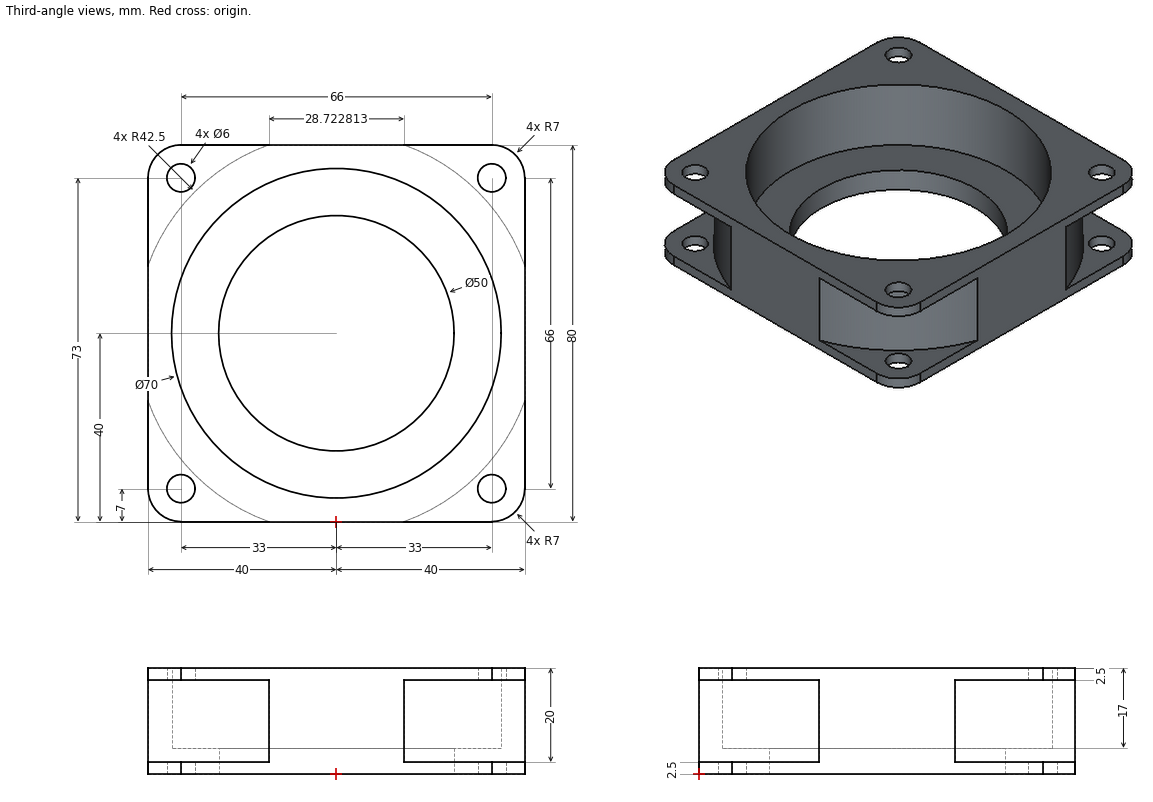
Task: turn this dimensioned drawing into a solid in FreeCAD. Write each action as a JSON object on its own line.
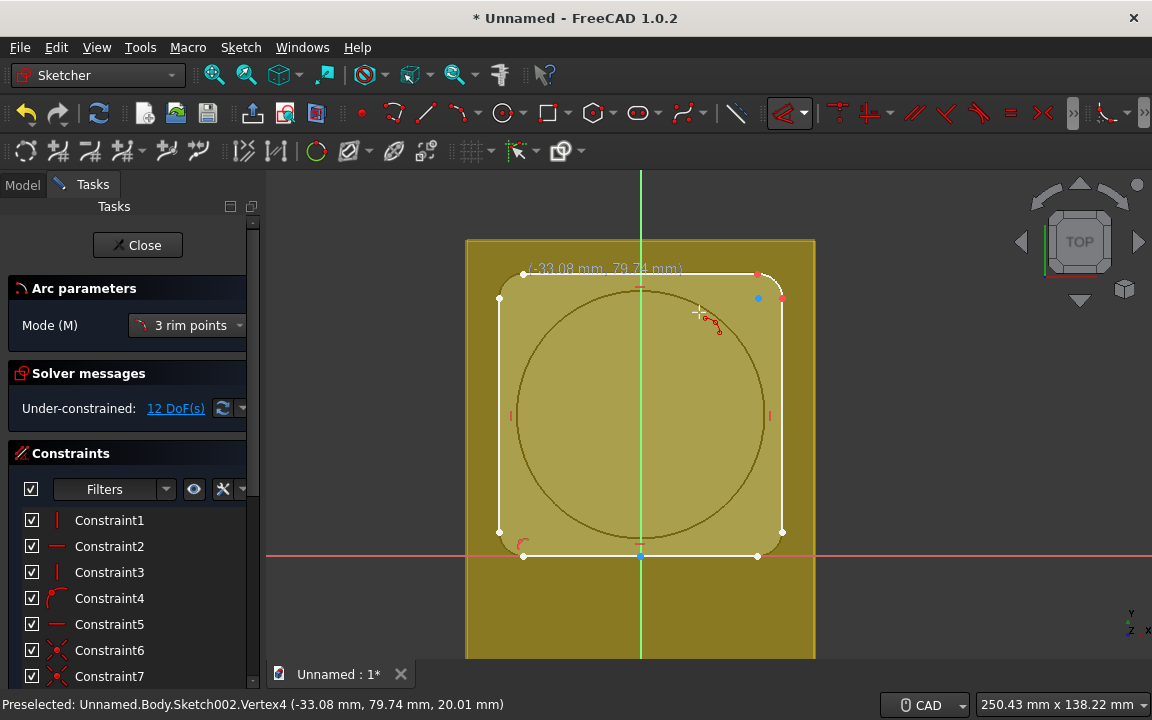
{"action": "left_click", "coordinate": [499, 299]}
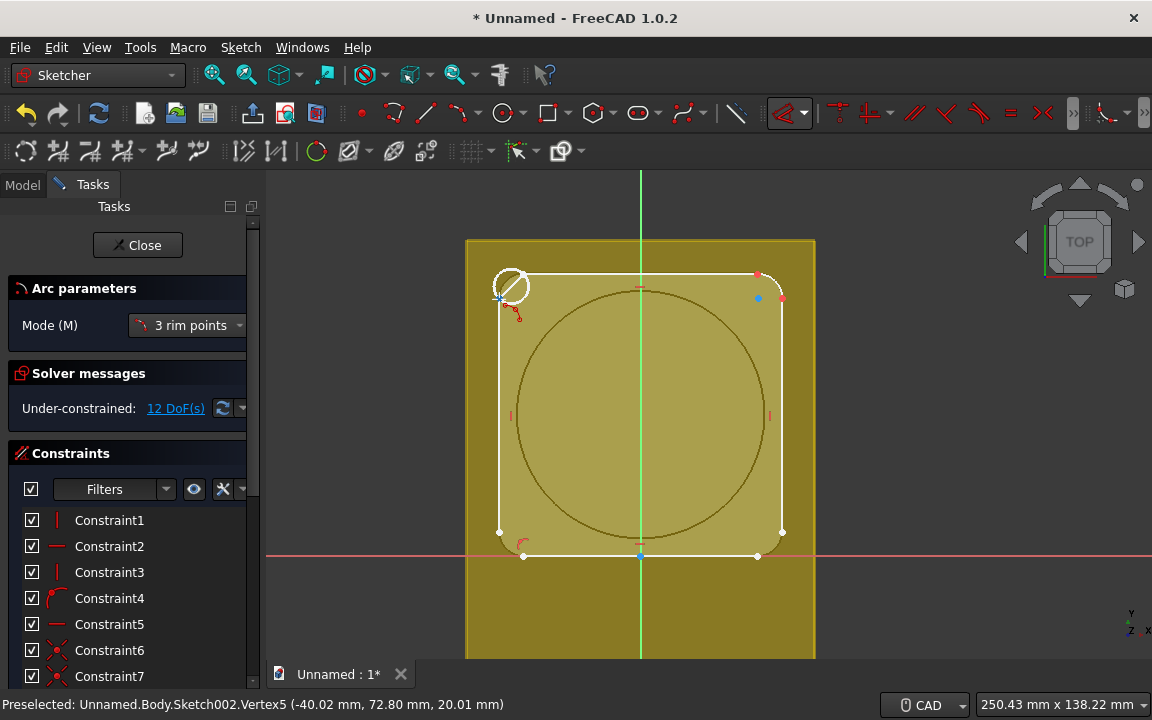
{"action": "scroll", "coordinate": [506, 280], "scroll_direction": "up", "scroll_amount": 4}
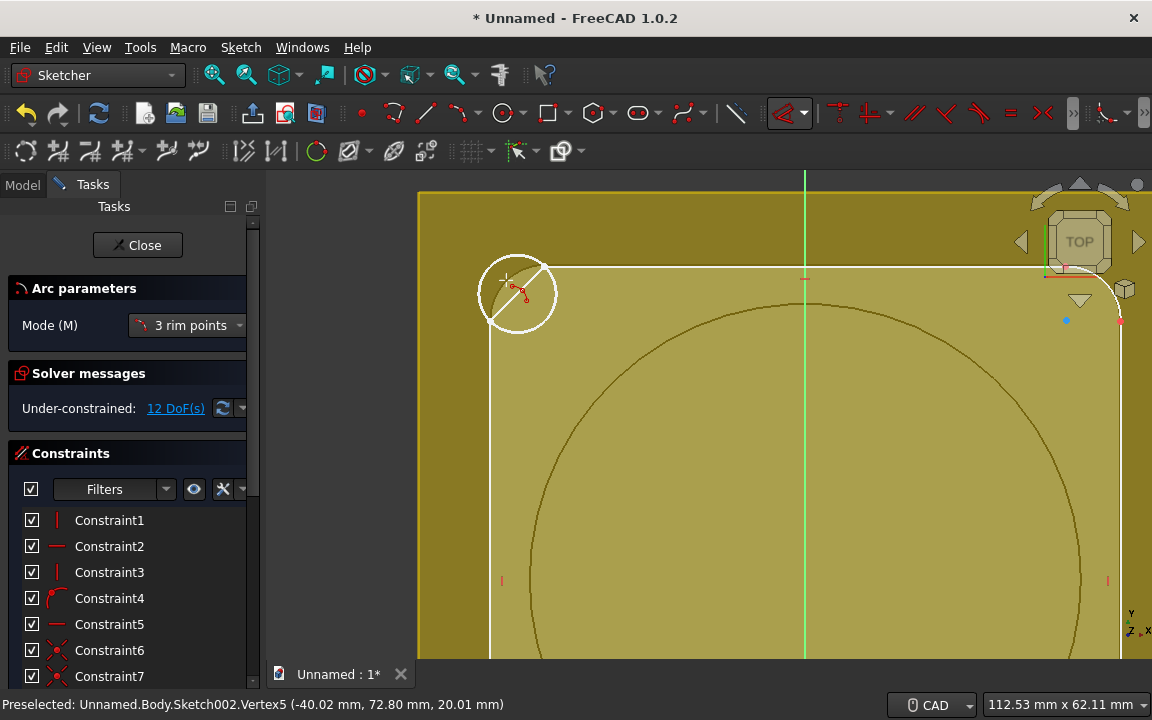
{"action": "left_click", "coordinate": [506, 281]}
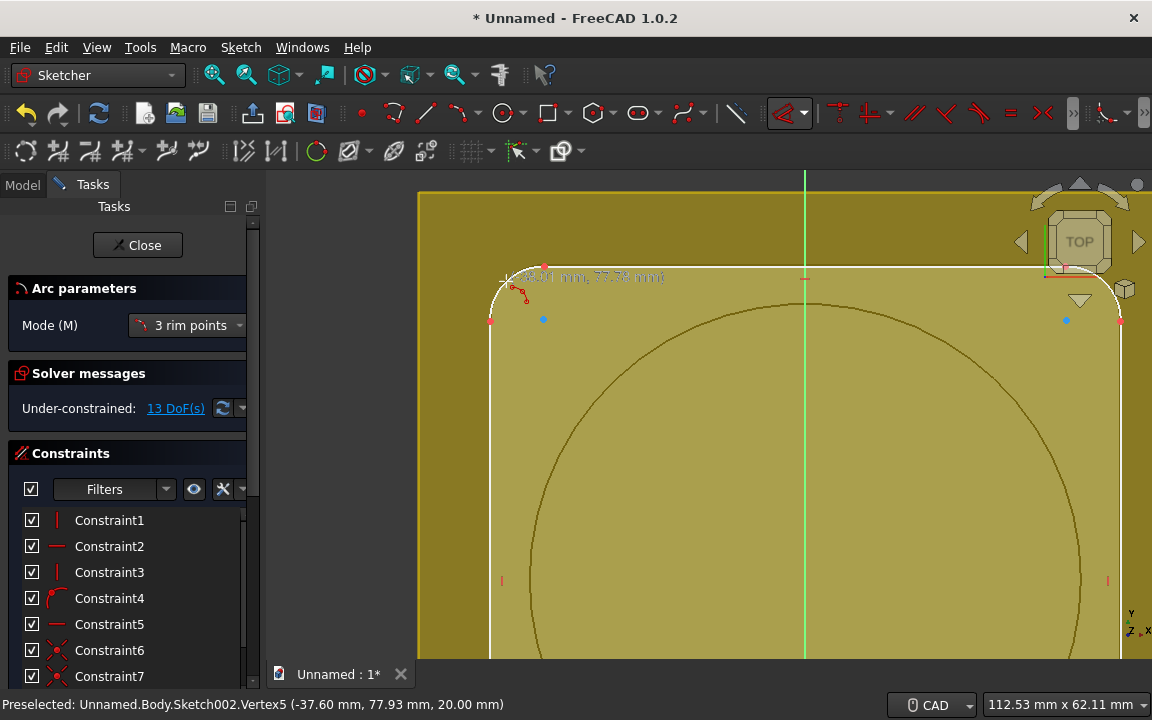
{"action": "scroll", "coordinate": [506, 280], "scroll_direction": "down", "scroll_amount": 4}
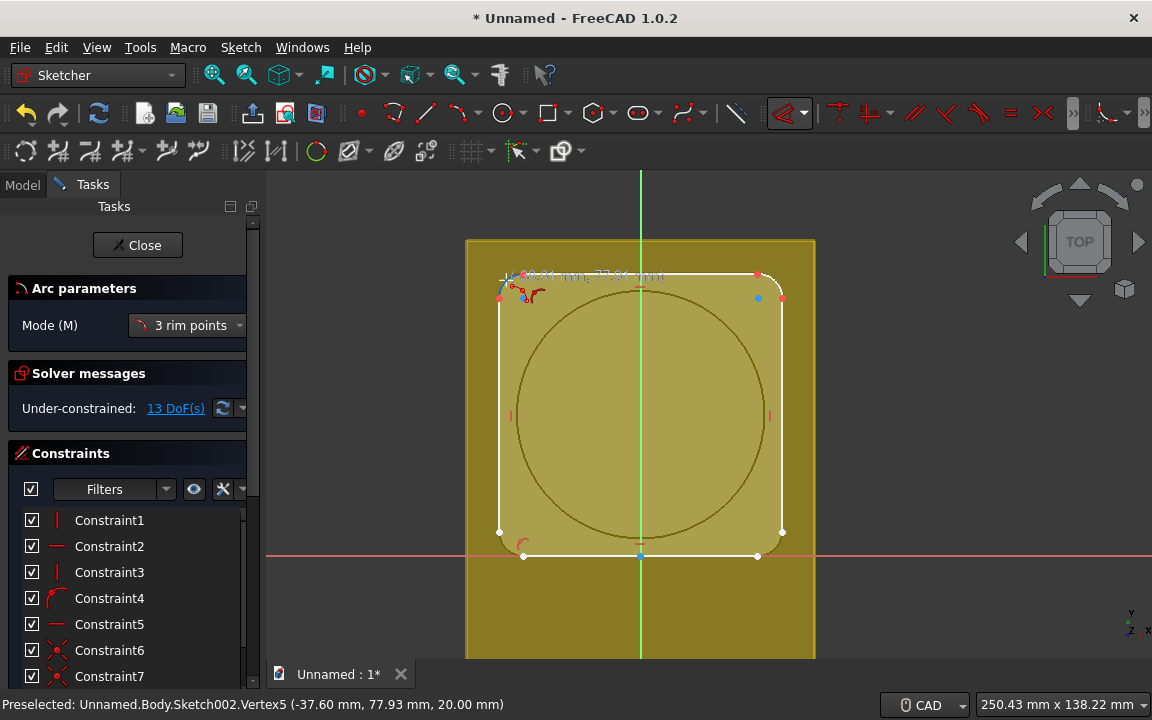
{"action": "left_click", "coordinate": [499, 532]}
{"action": "left_click", "coordinate": [524, 556]}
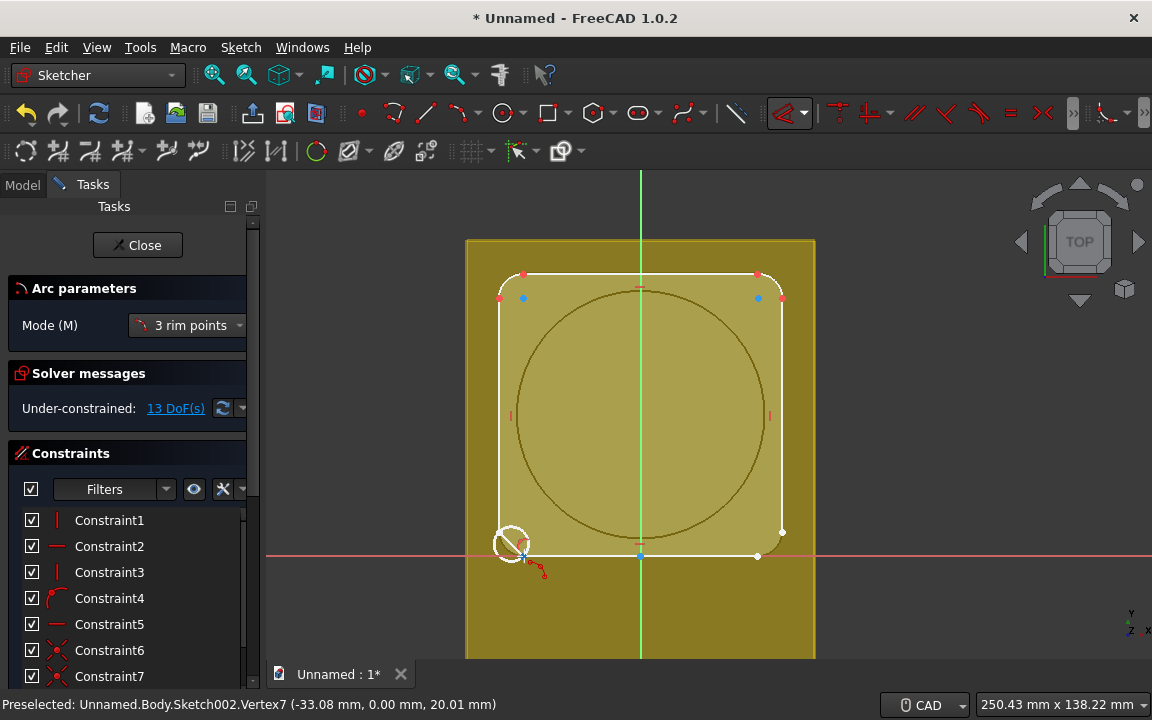
{"action": "scroll", "coordinate": [506, 549], "scroll_direction": "up", "scroll_amount": 4}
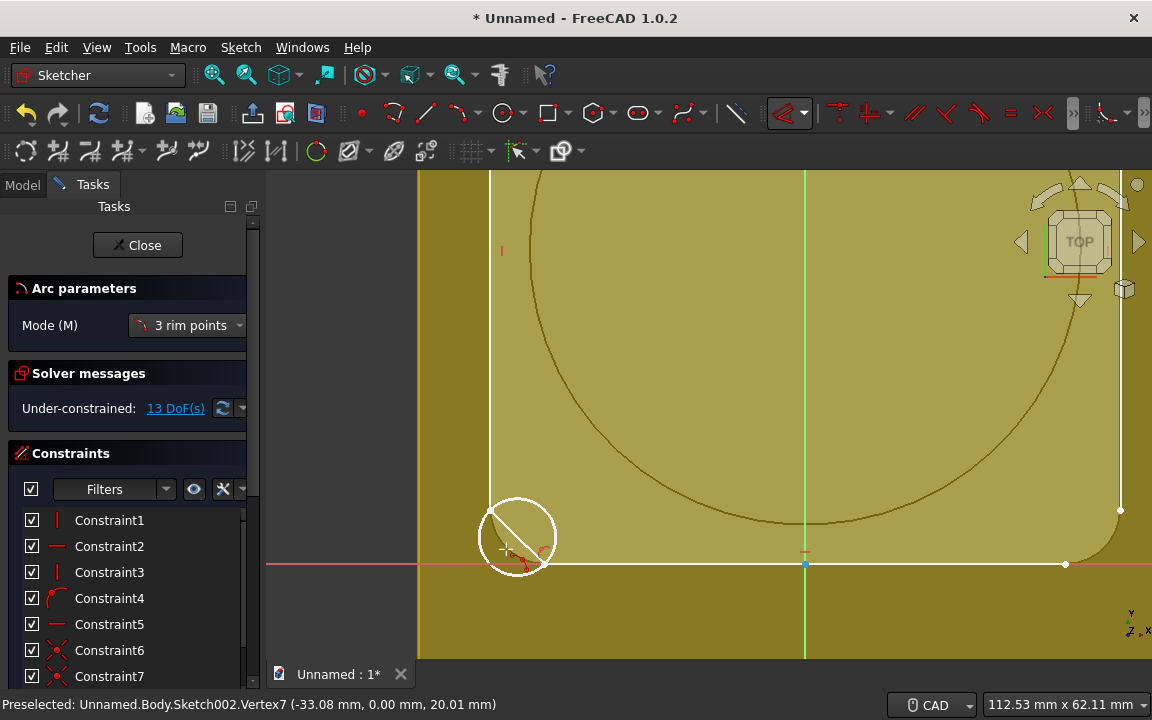
{"action": "left_click", "coordinate": [506, 548]}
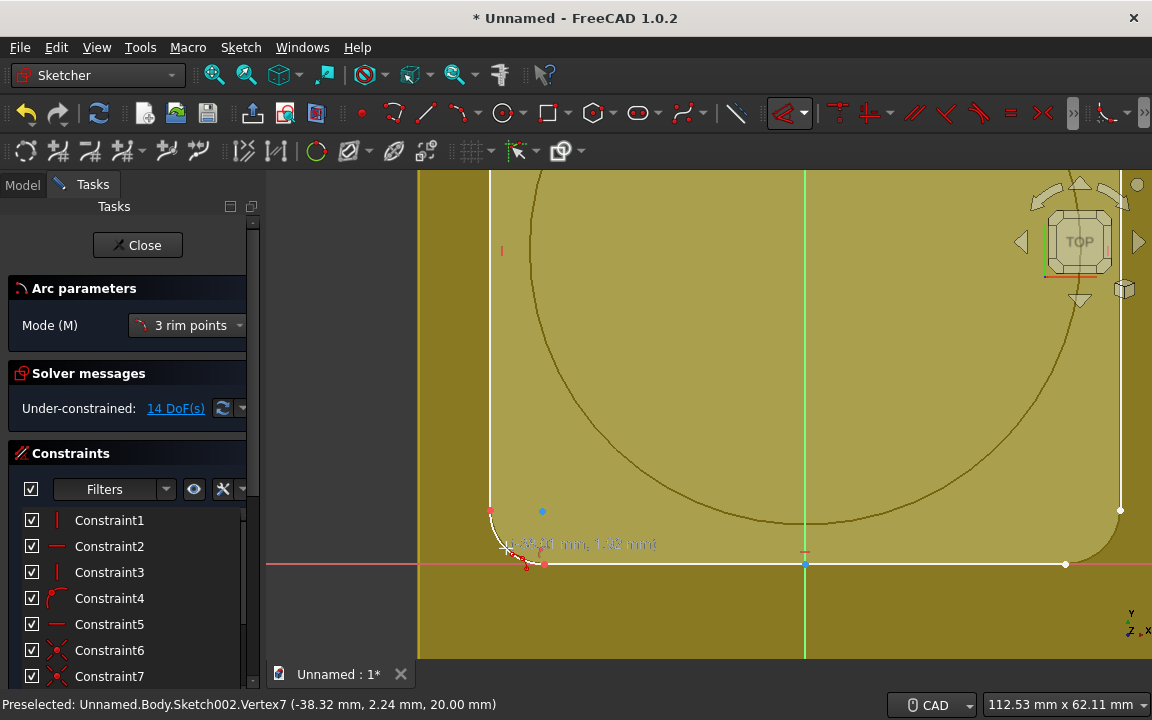
{"action": "scroll", "coordinate": [506, 549], "scroll_direction": "down", "scroll_amount": 4}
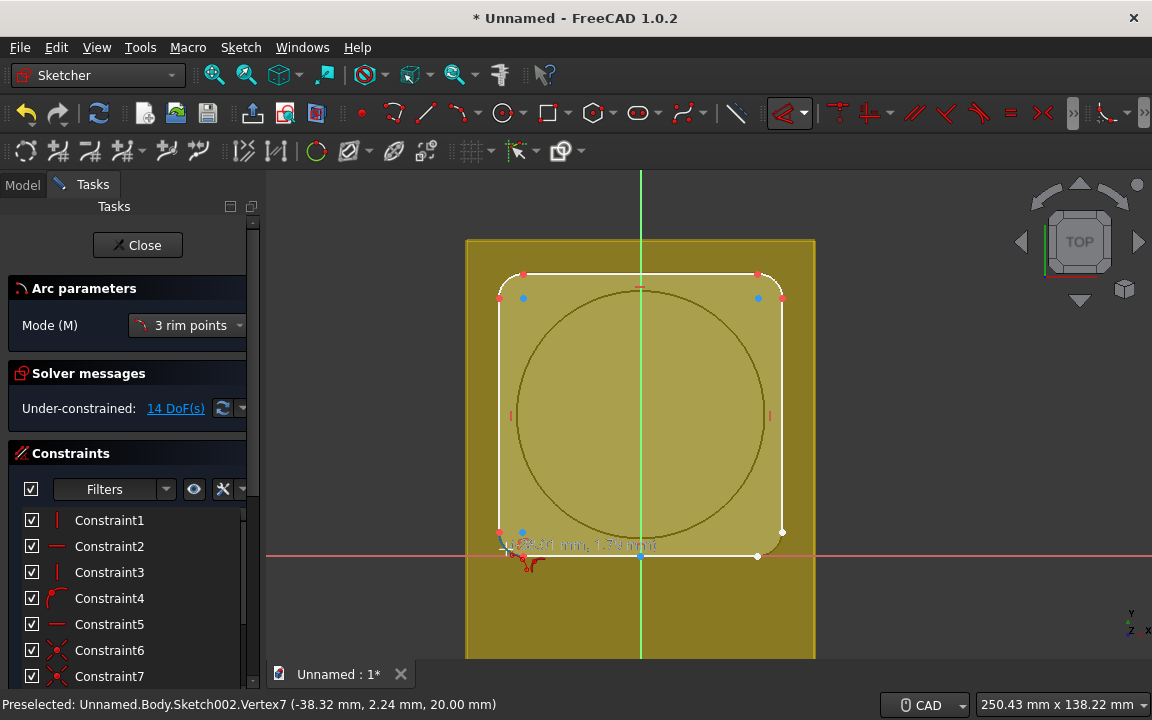
{"action": "left_click", "coordinate": [758, 556]}
{"action": "left_click", "coordinate": [782, 532]}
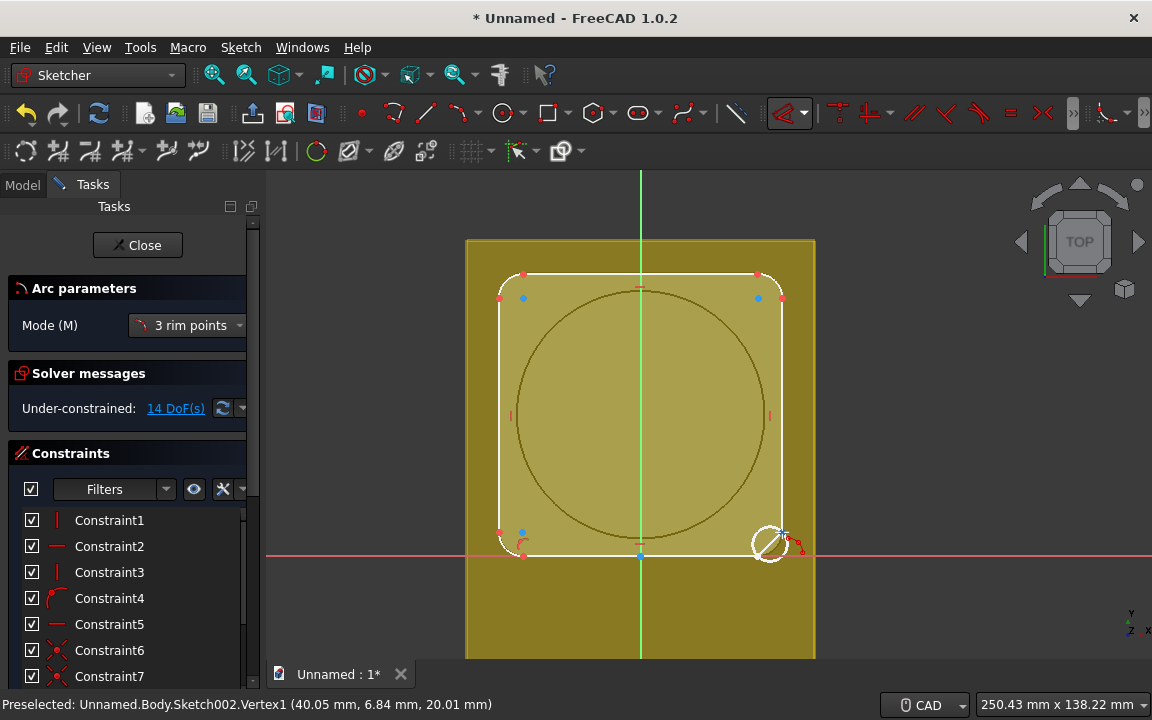
{"action": "scroll", "coordinate": [775, 549], "scroll_direction": "up", "scroll_amount": 4}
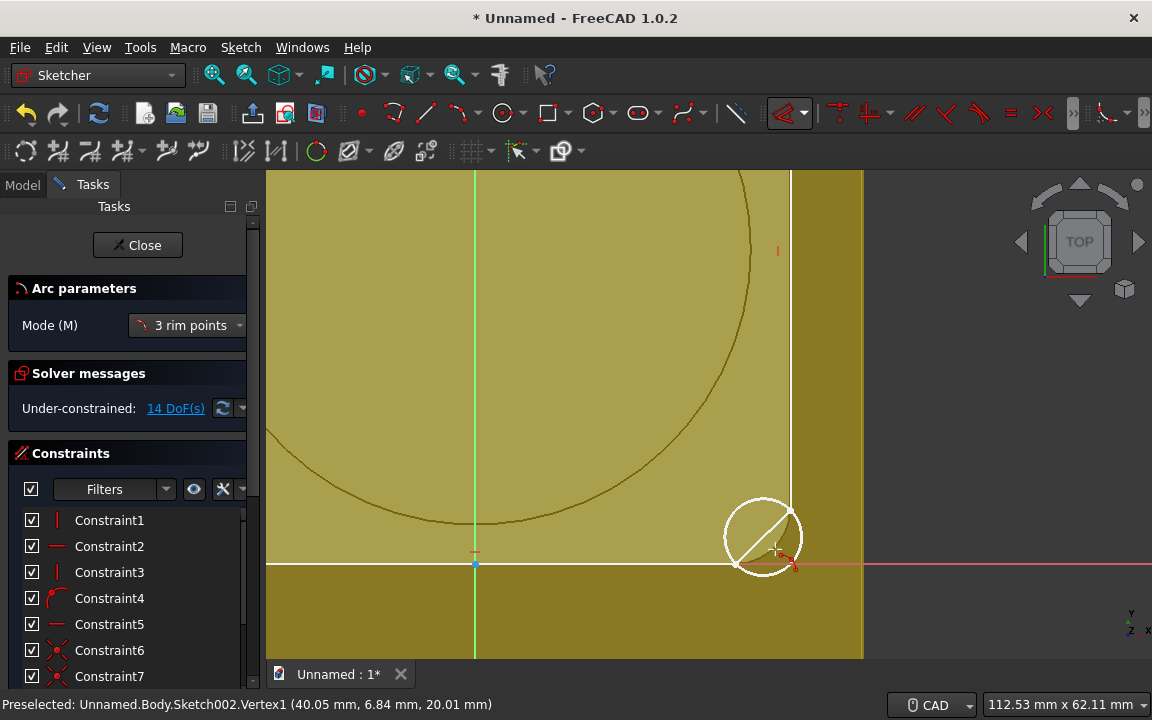
{"action": "left_click", "coordinate": [774, 548]}
{"action": "key", "text": "Escape"}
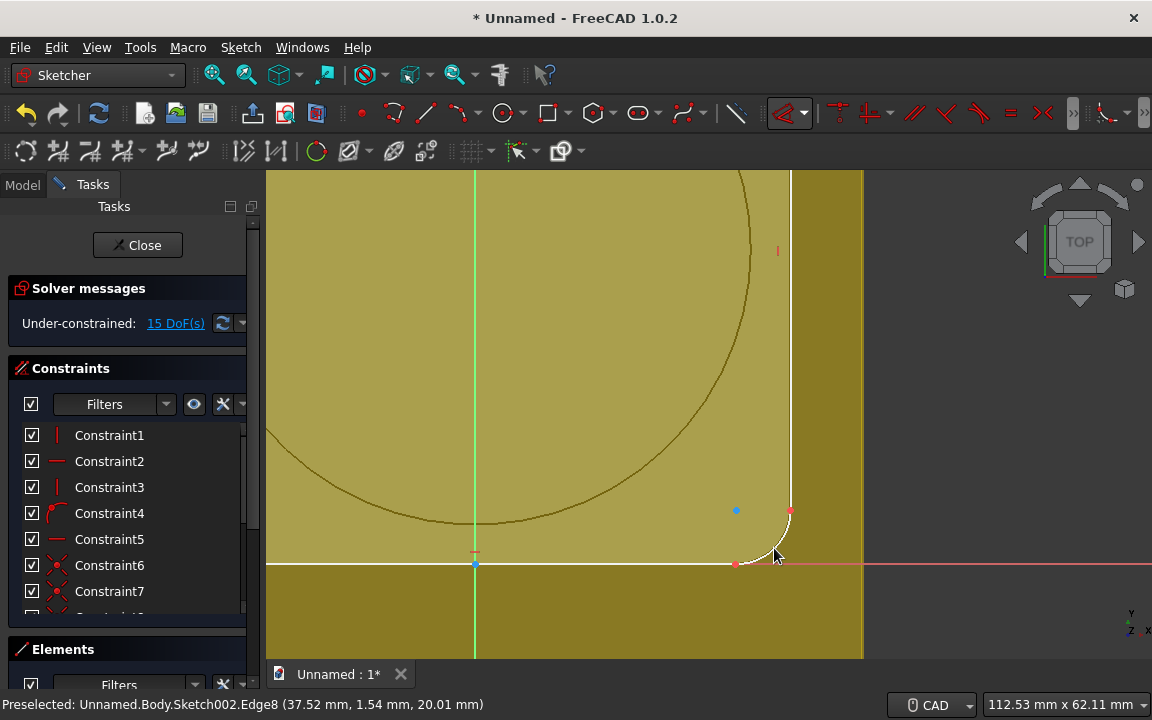
{"action": "left_click", "coordinate": [791, 354]}